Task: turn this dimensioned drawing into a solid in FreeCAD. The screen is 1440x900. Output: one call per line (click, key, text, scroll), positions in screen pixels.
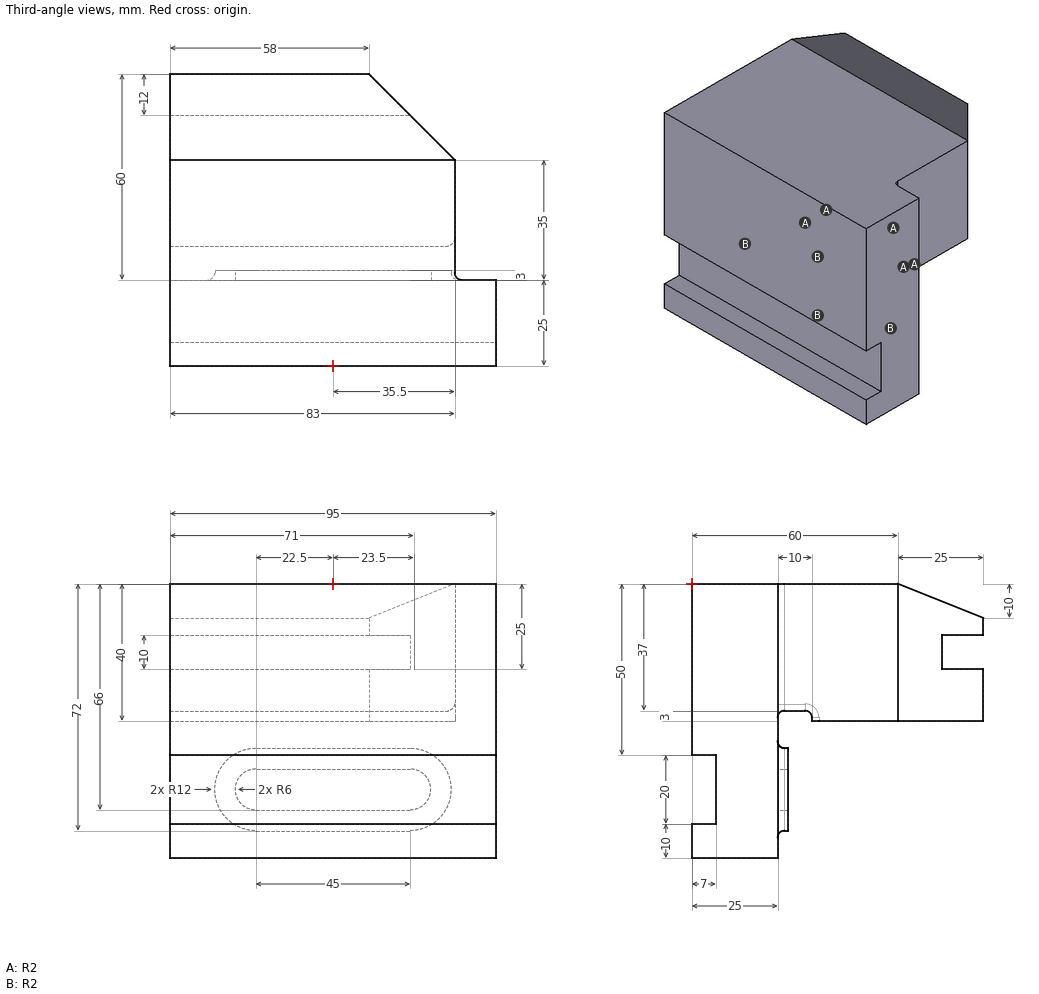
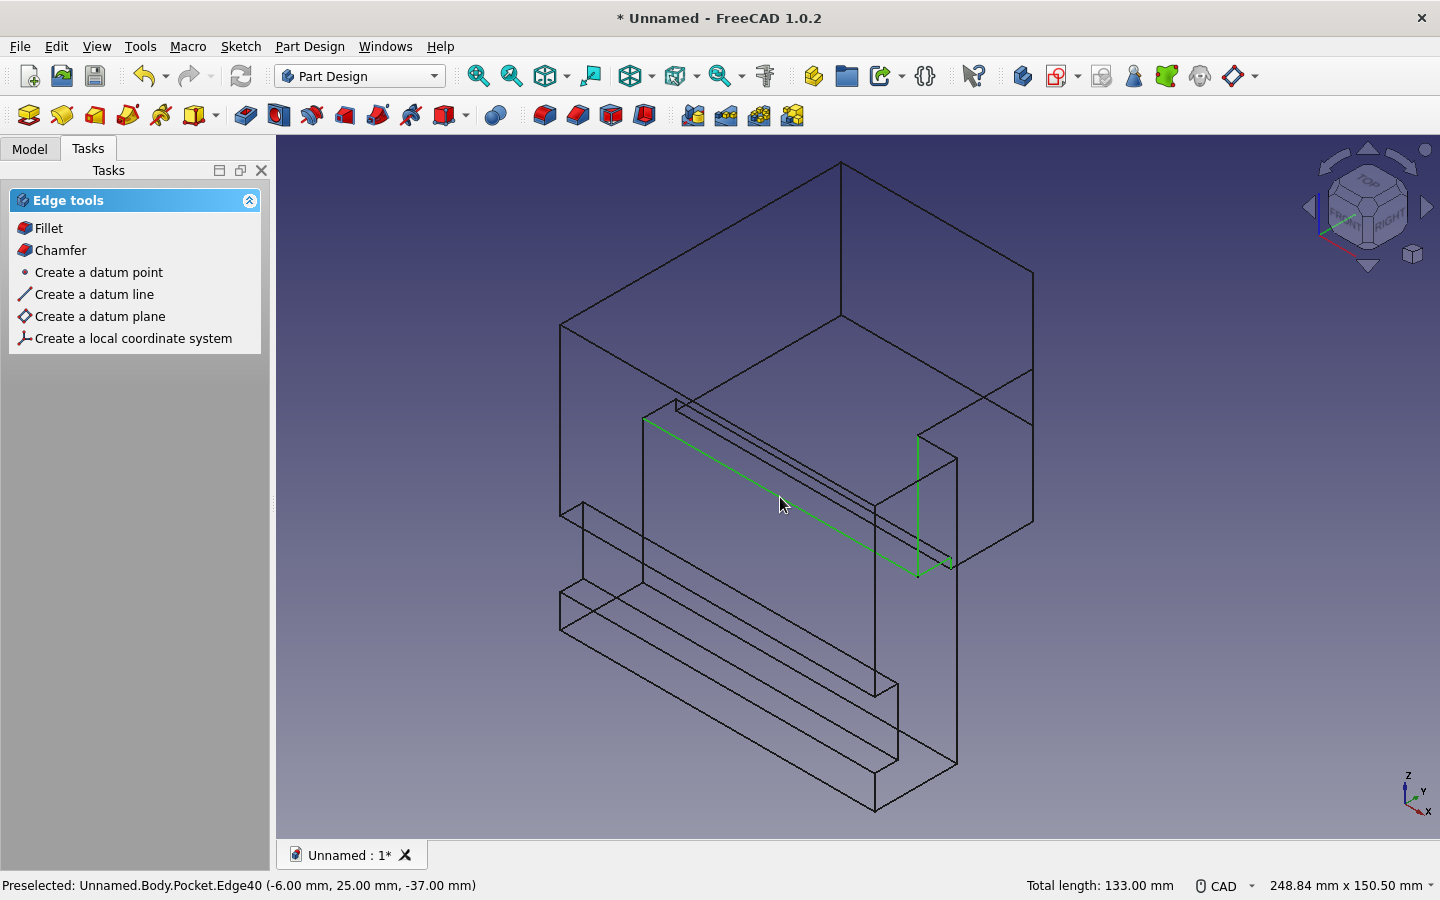
click(813, 477, ctrl)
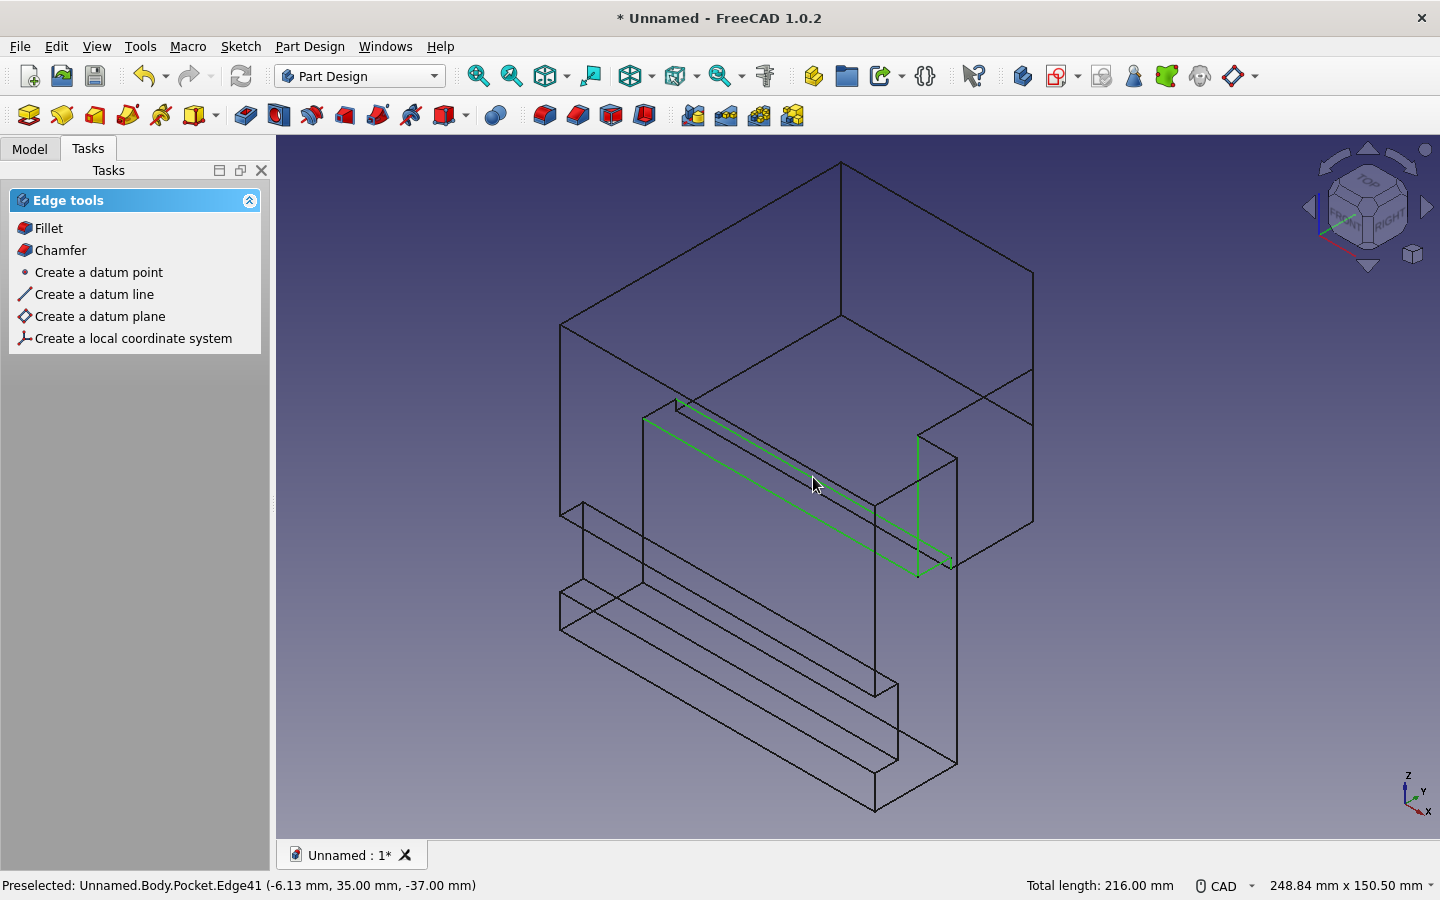
key(v)
key(1)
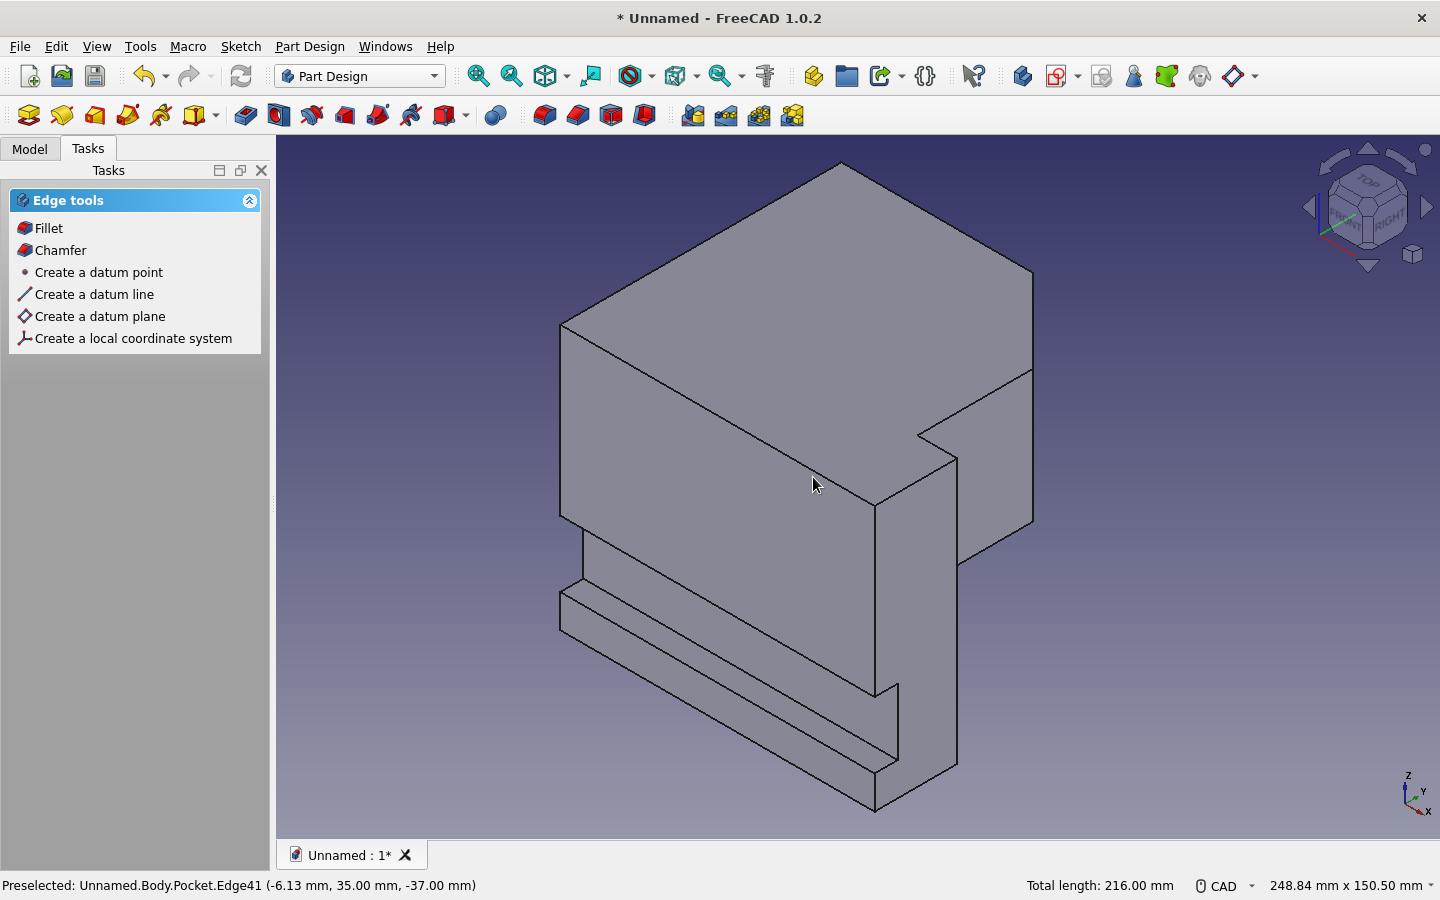
click(545, 116)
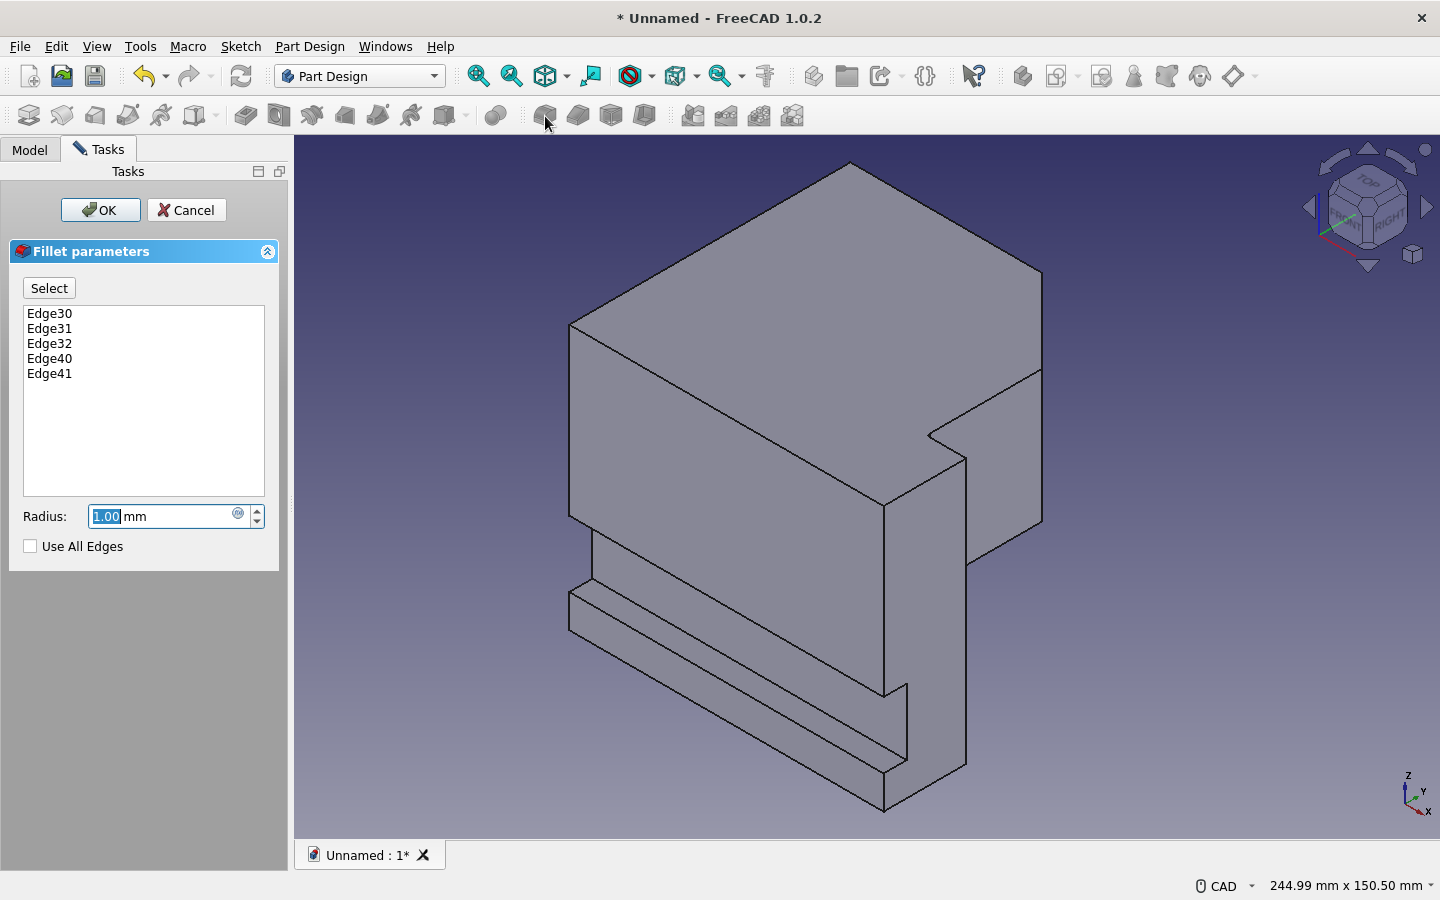
text(2)
key(Tab)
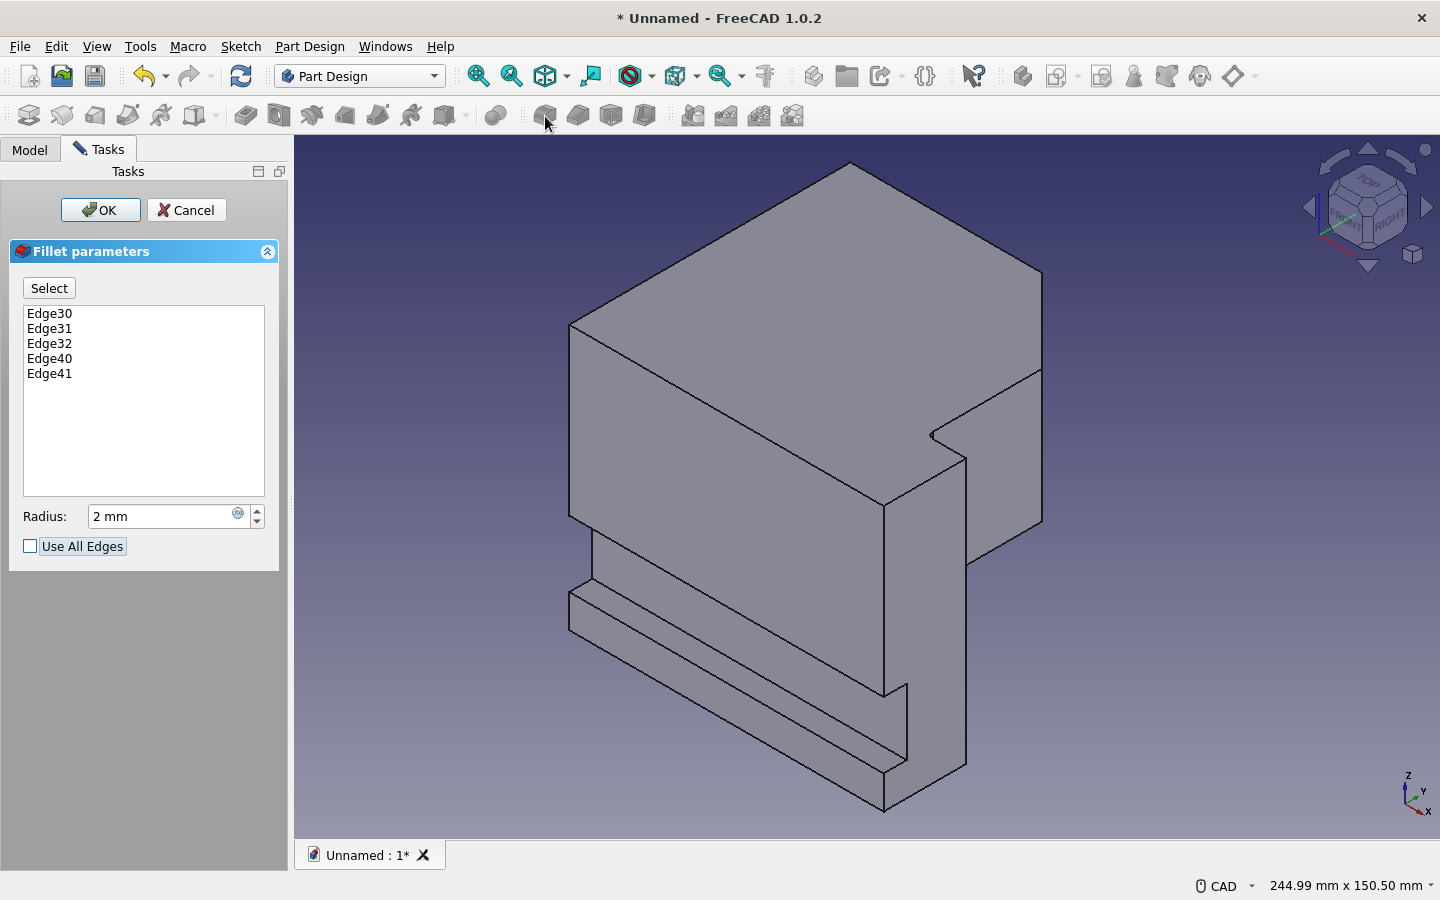
click(101, 210)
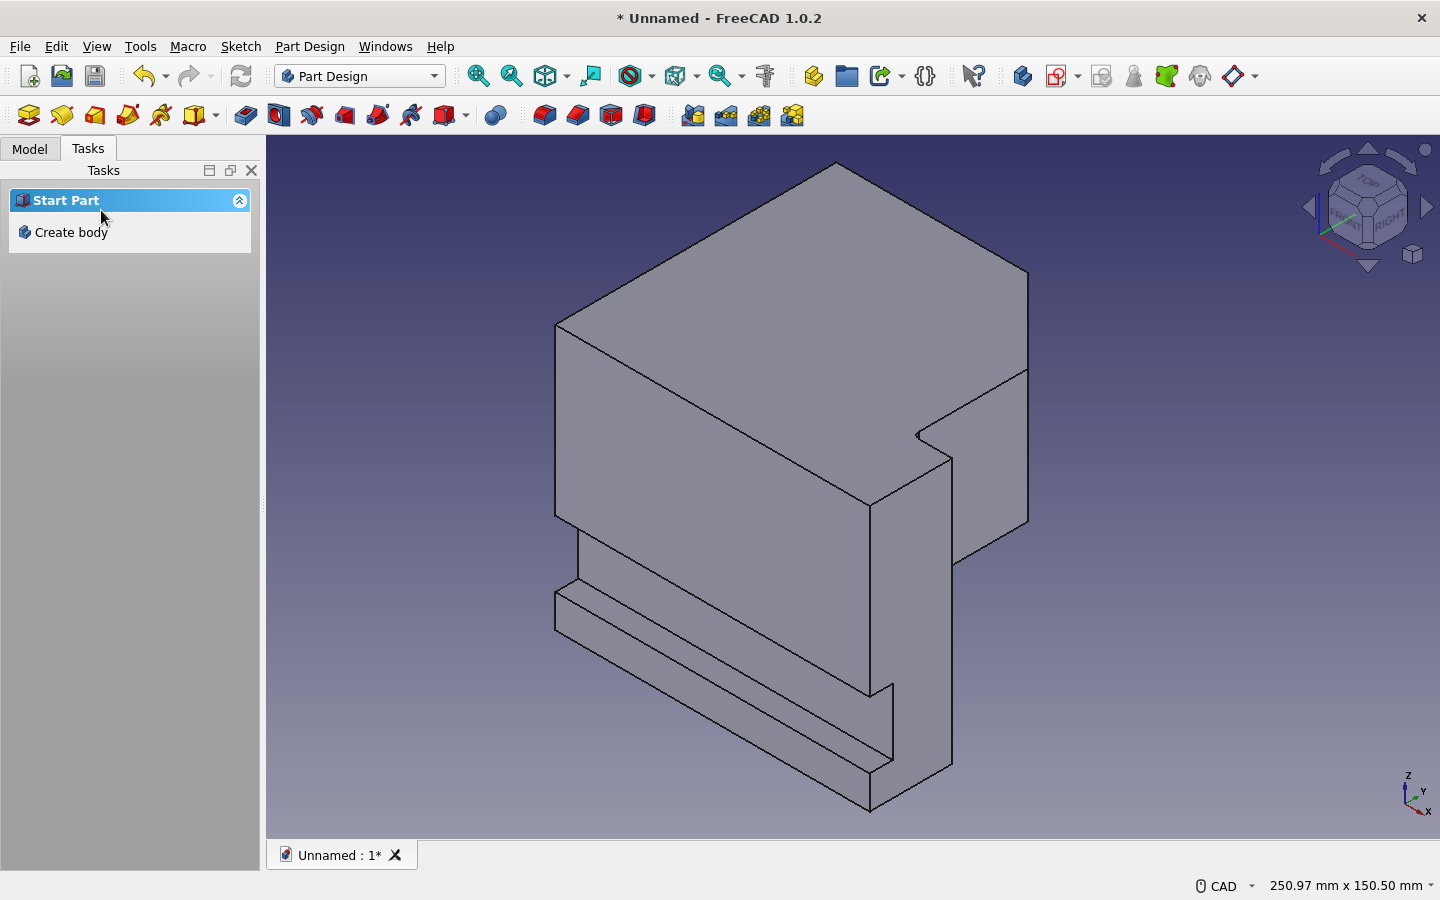
key(4)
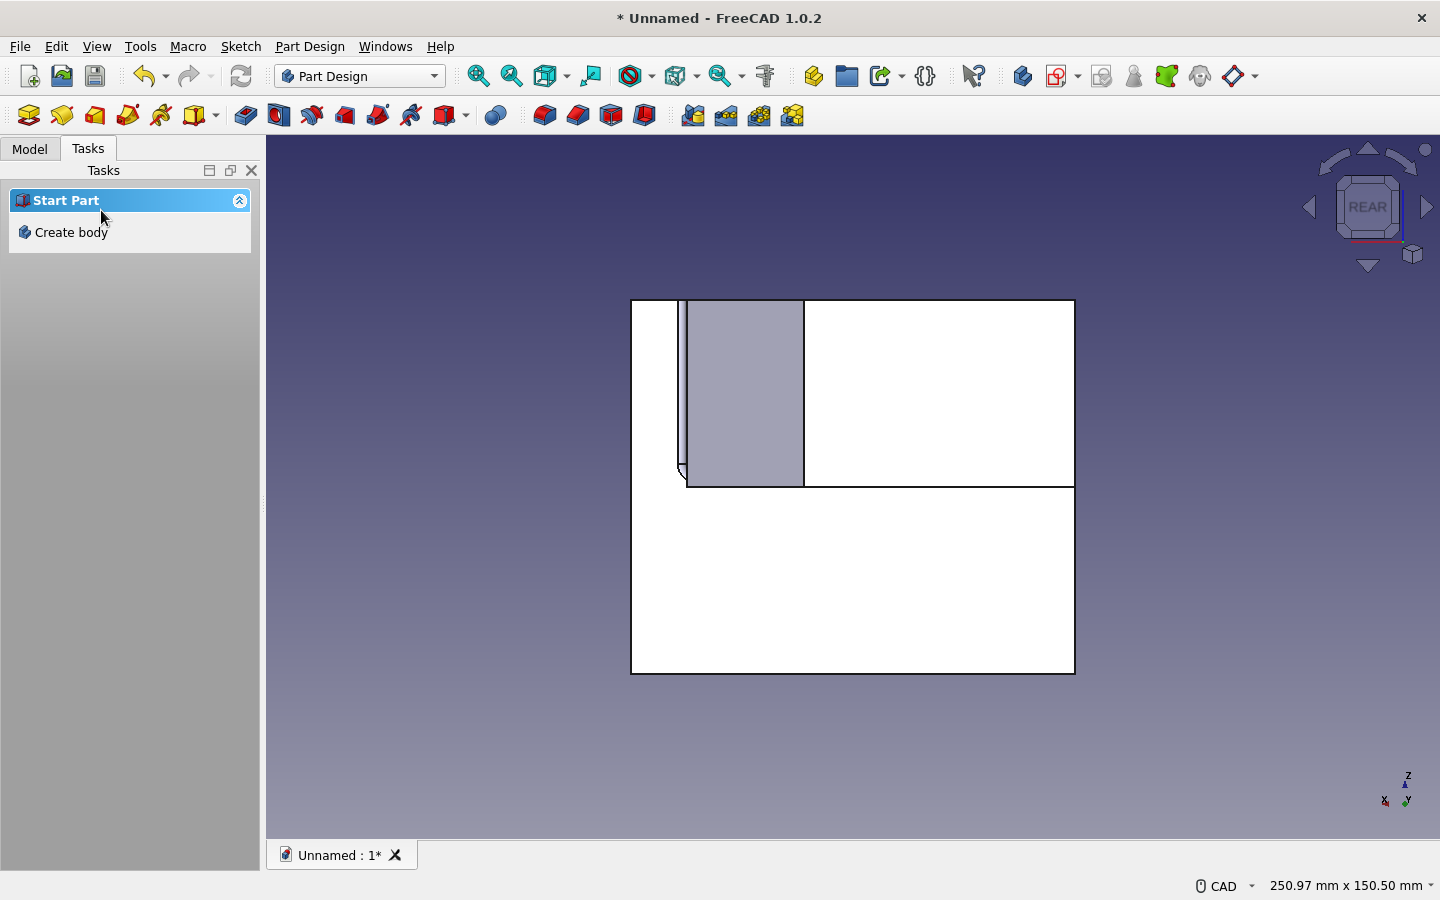
click(901, 392)